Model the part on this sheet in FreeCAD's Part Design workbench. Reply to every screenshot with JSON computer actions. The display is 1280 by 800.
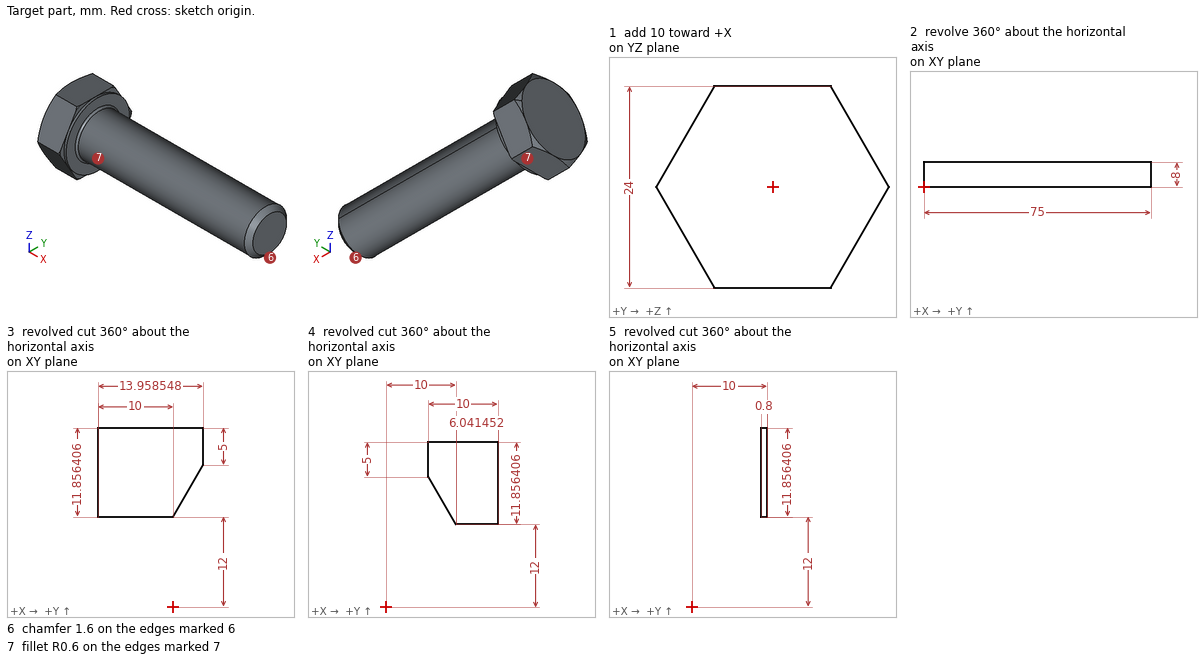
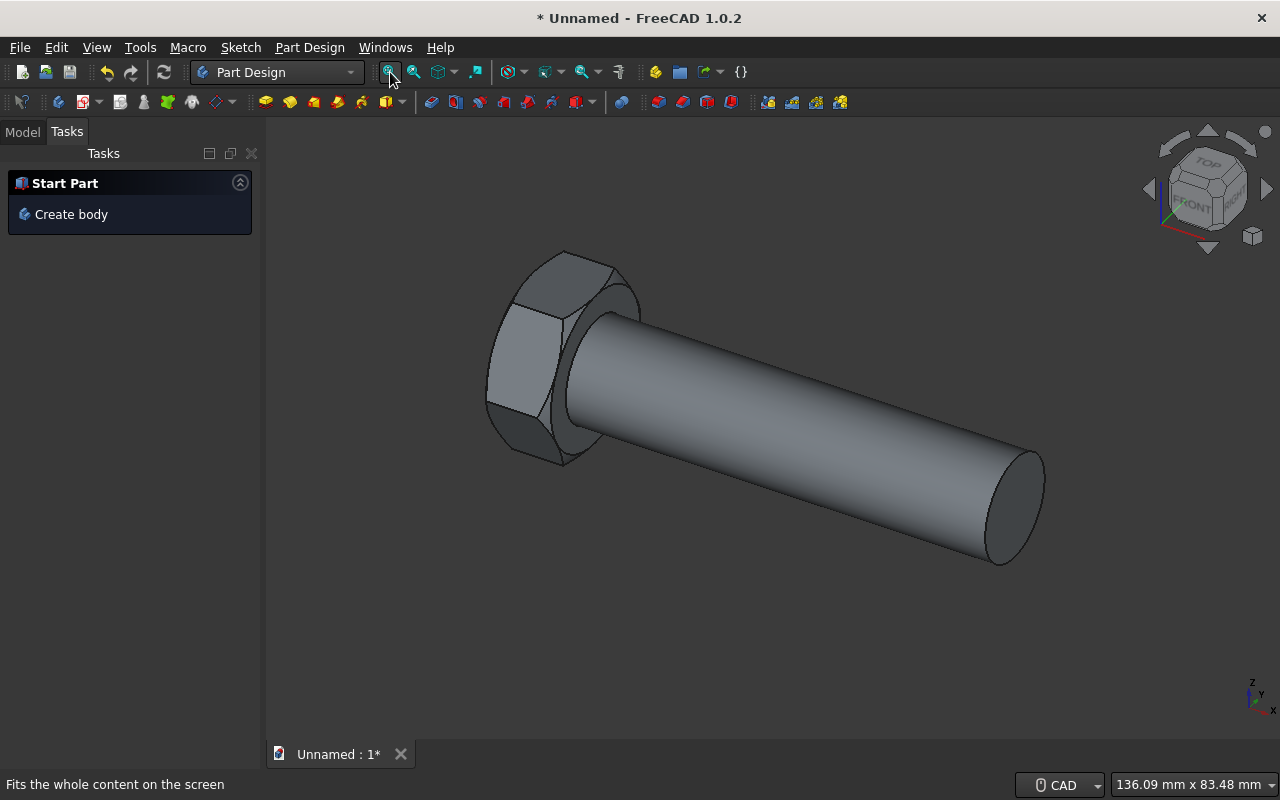
{"action": "left_click", "coordinate": [84, 102]}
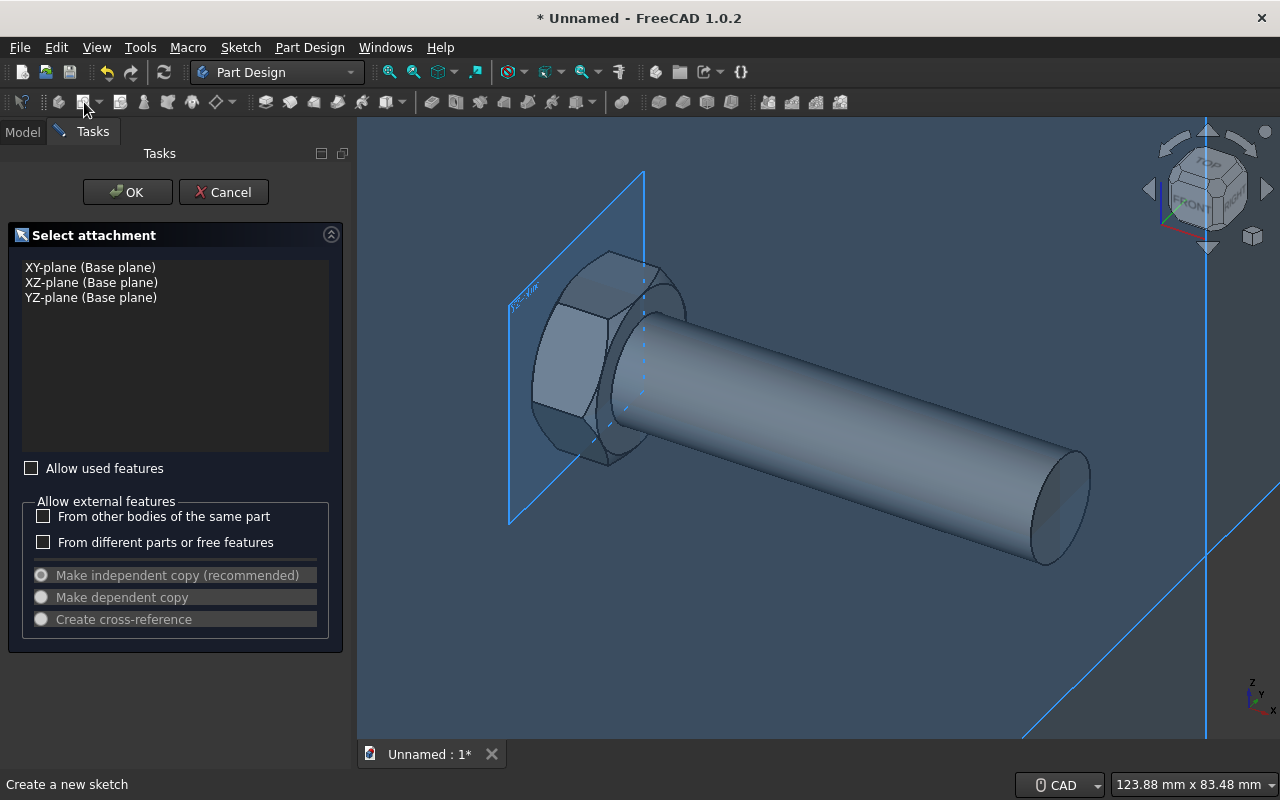
{"action": "left_click", "coordinate": [82, 268]}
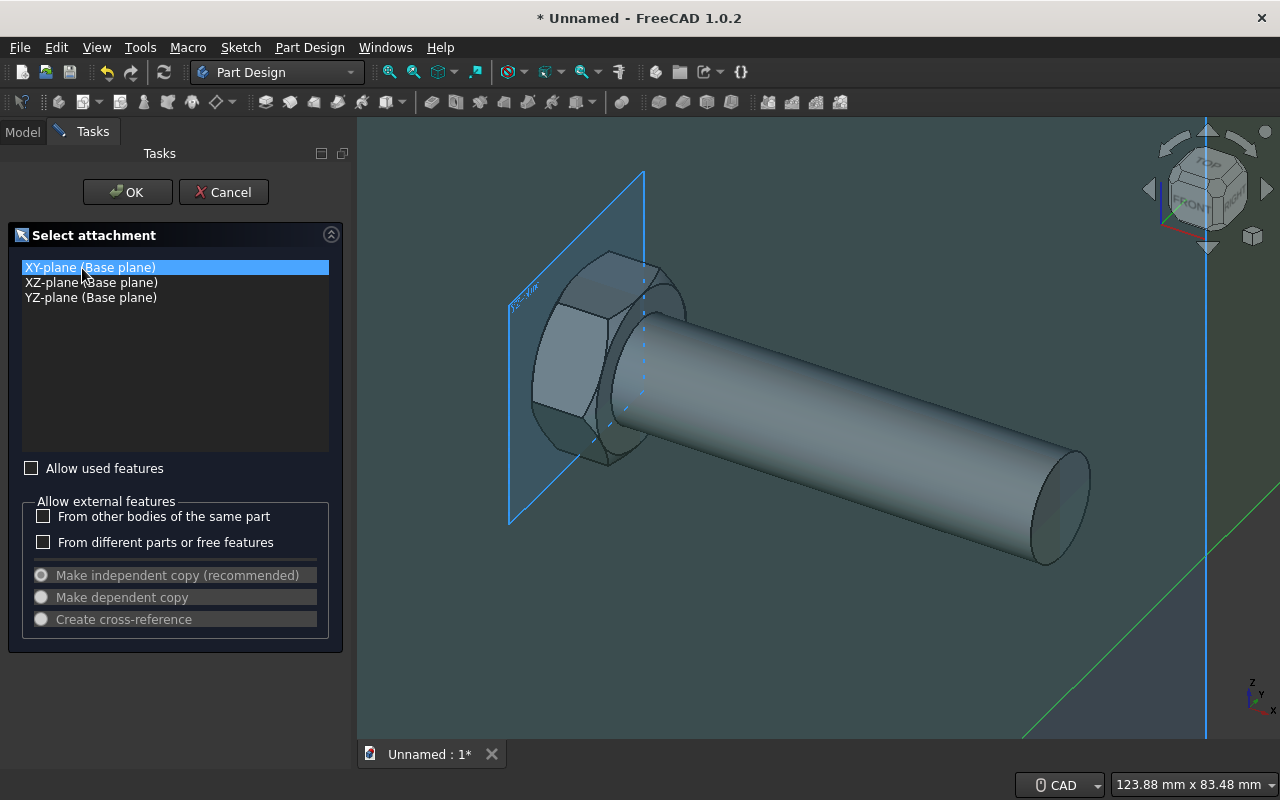
{"action": "left_click", "coordinate": [128, 192]}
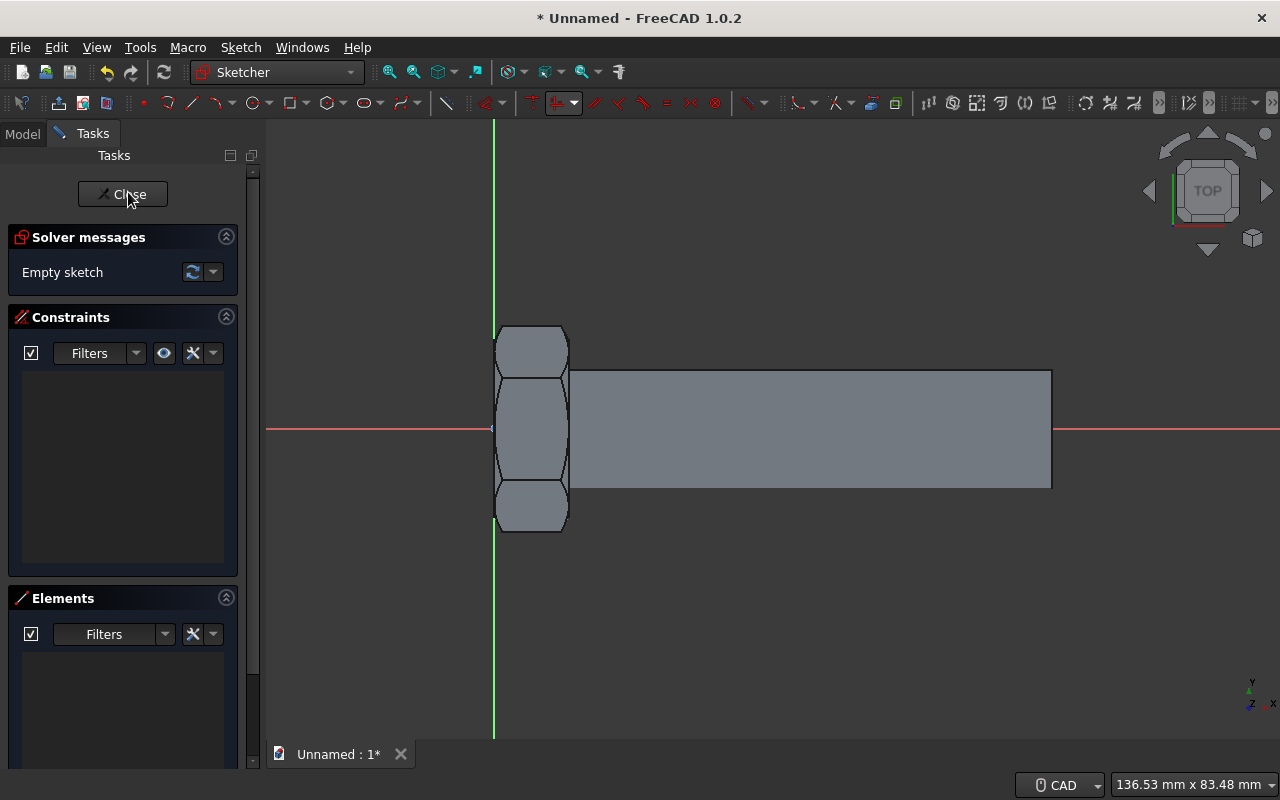
{"action": "left_click", "coordinate": [108, 104]}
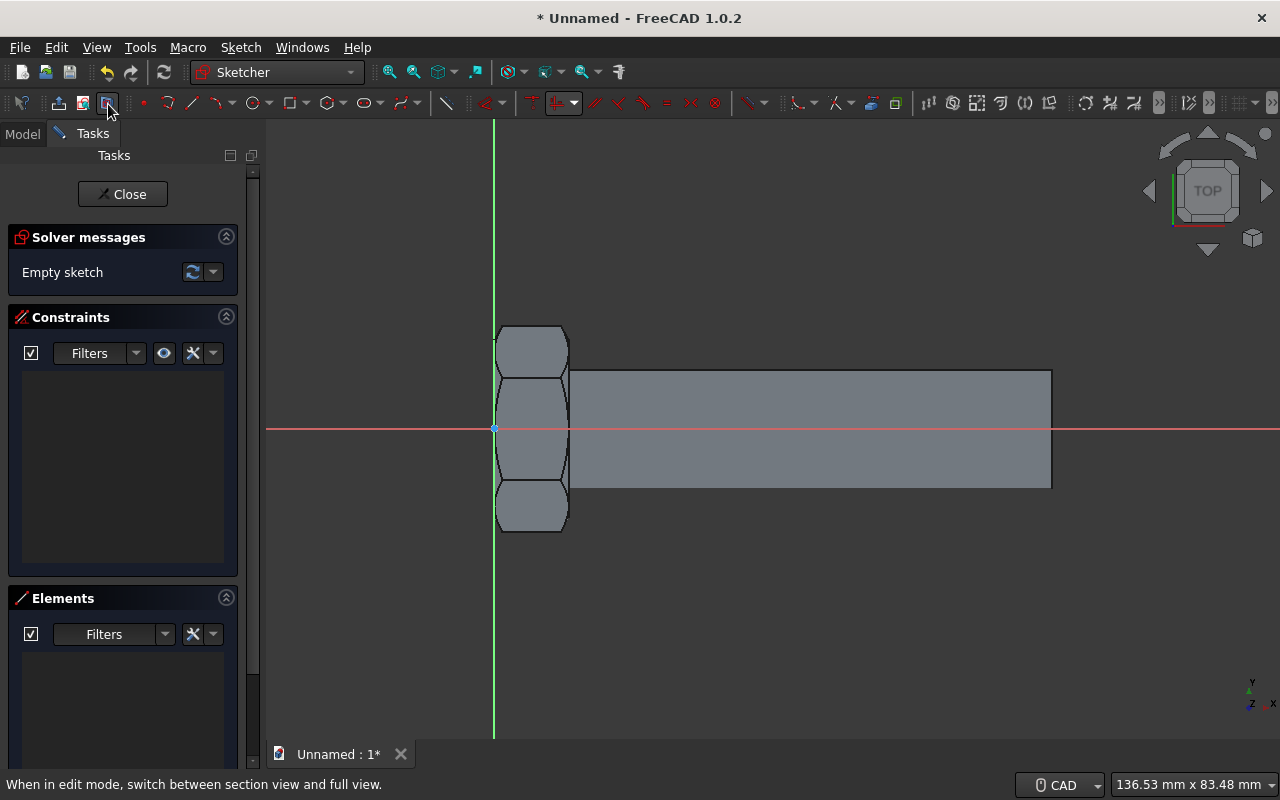
{"action": "scroll", "coordinate": [391, 268], "scroll_direction": "up", "scroll_amount": 4}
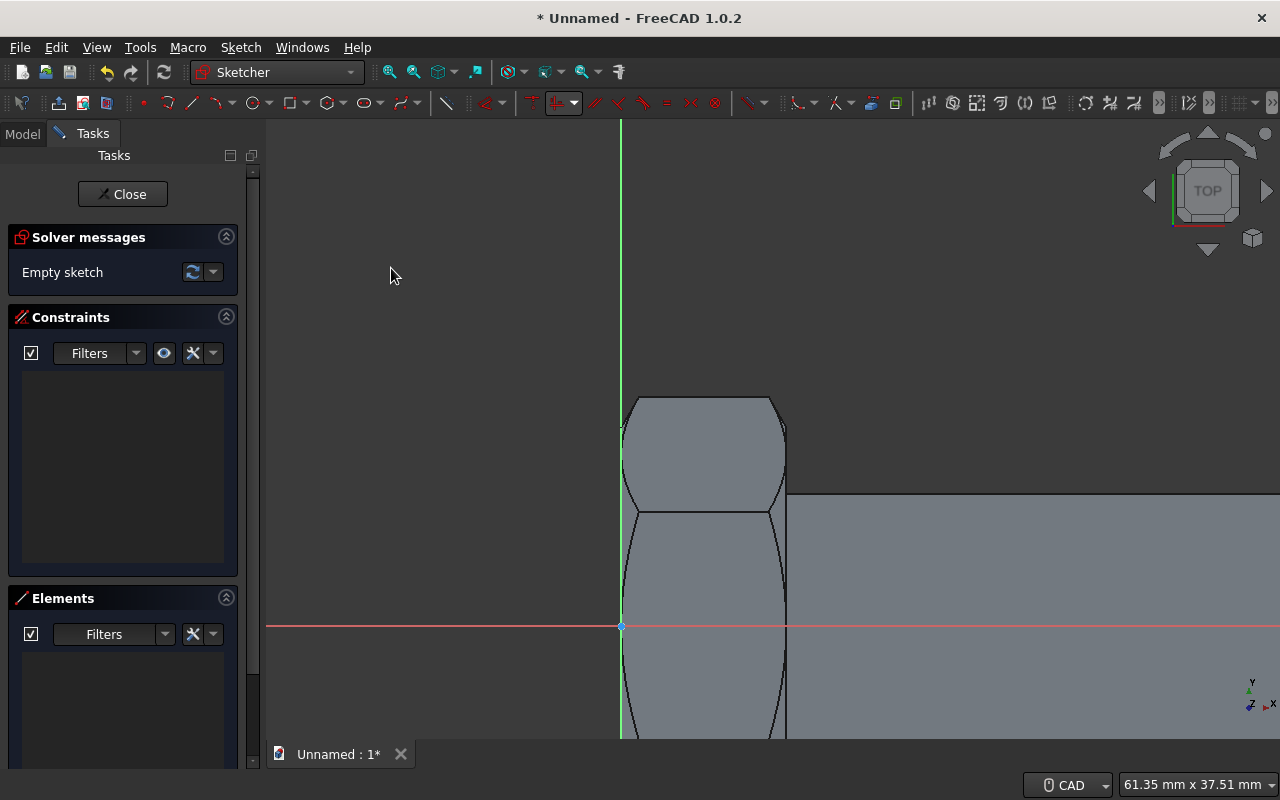
{"action": "left_click", "coordinate": [290, 104]}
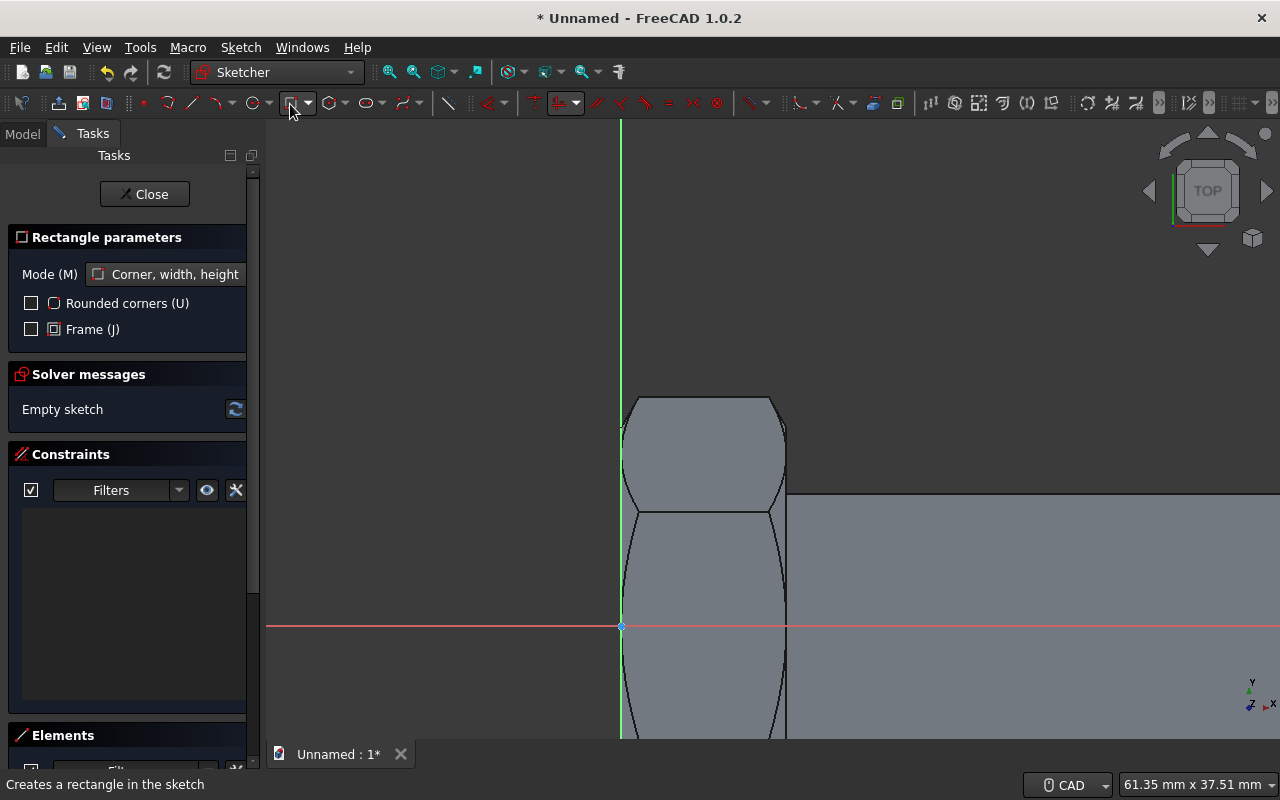
{"action": "left_click", "coordinate": [773, 232]}
{"action": "mouse_move", "coordinate": [786, 428]}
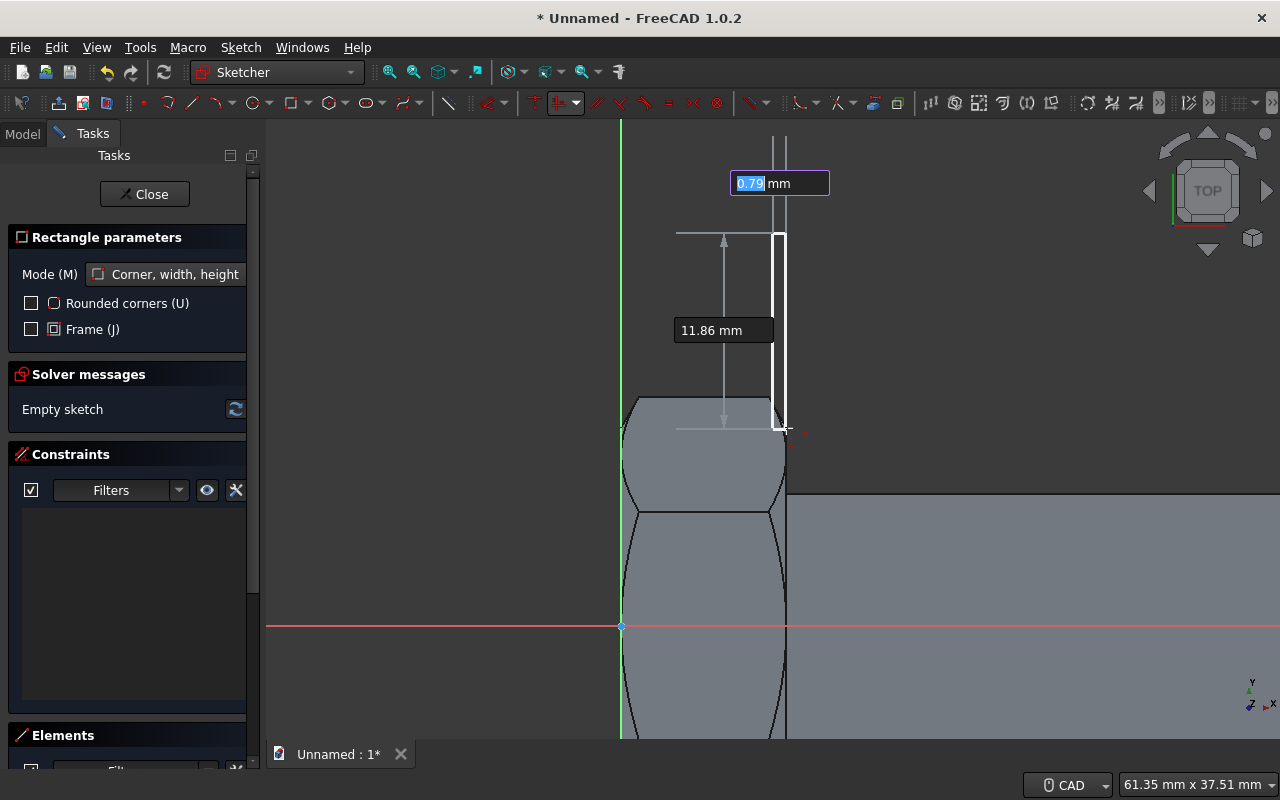
{"action": "type", "text": "0.8"}
{"action": "key", "text": "Tab"}
{"action": "type", "text": "11.856406"}
{"action": "key", "text": "Return"}
{"action": "key", "text": "Escape"}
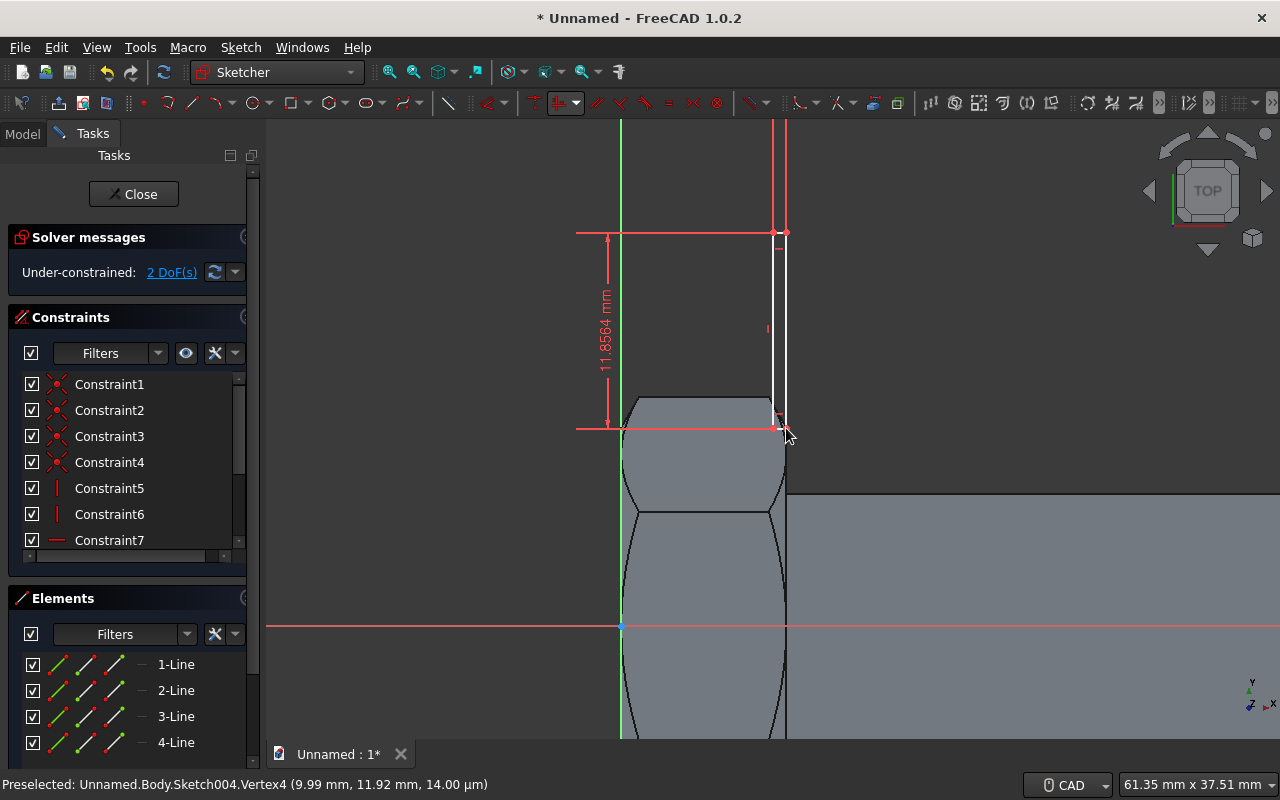
{"action": "left_click", "coordinate": [488, 104]}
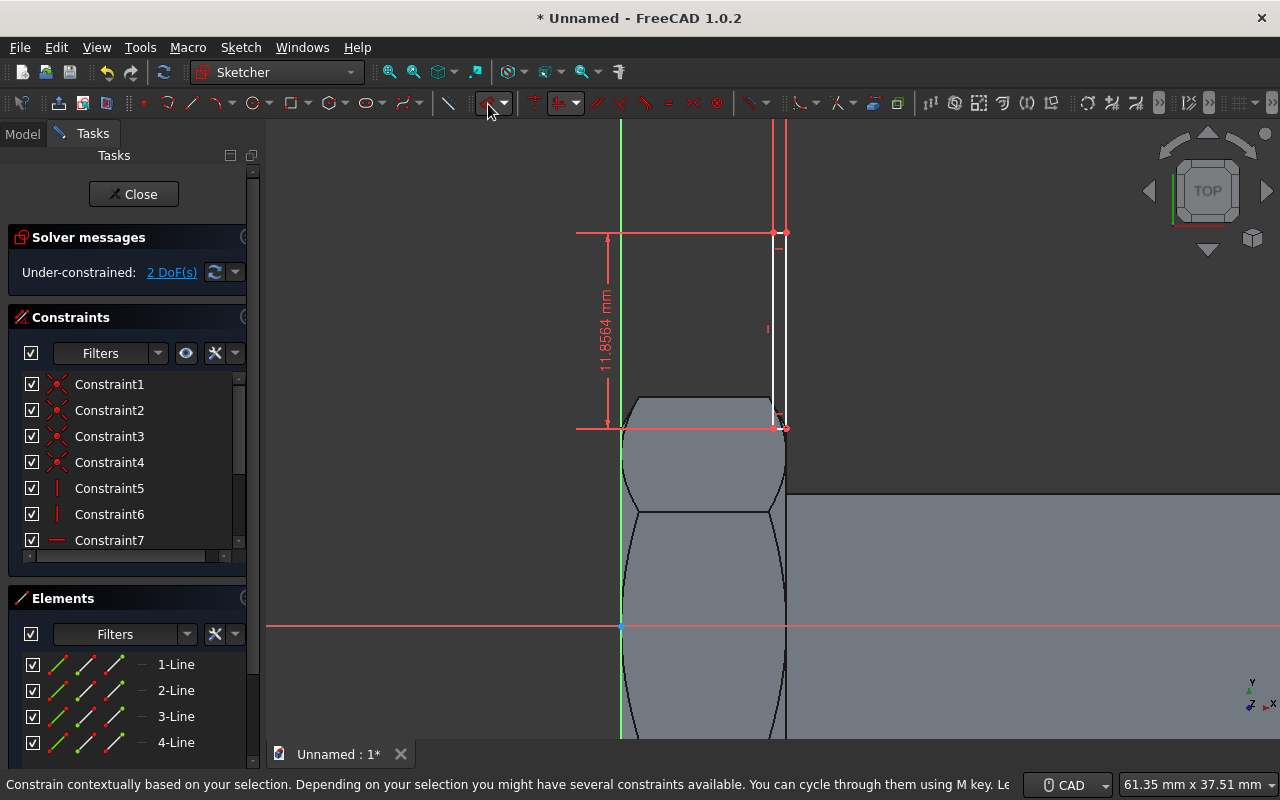
{"action": "left_click", "coordinate": [773, 429]}
{"action": "left_click", "coordinate": [587, 527]}